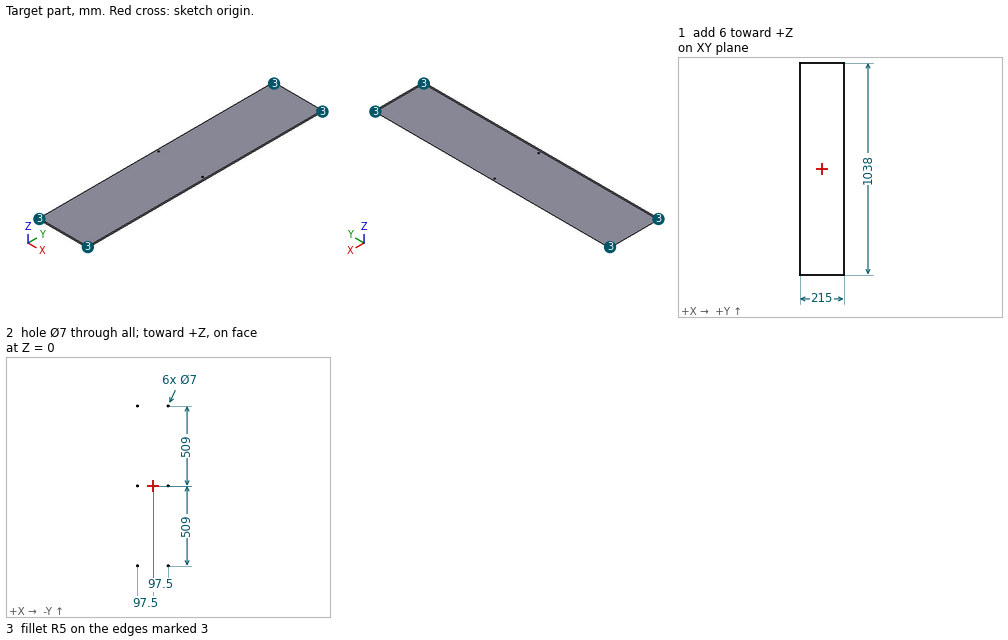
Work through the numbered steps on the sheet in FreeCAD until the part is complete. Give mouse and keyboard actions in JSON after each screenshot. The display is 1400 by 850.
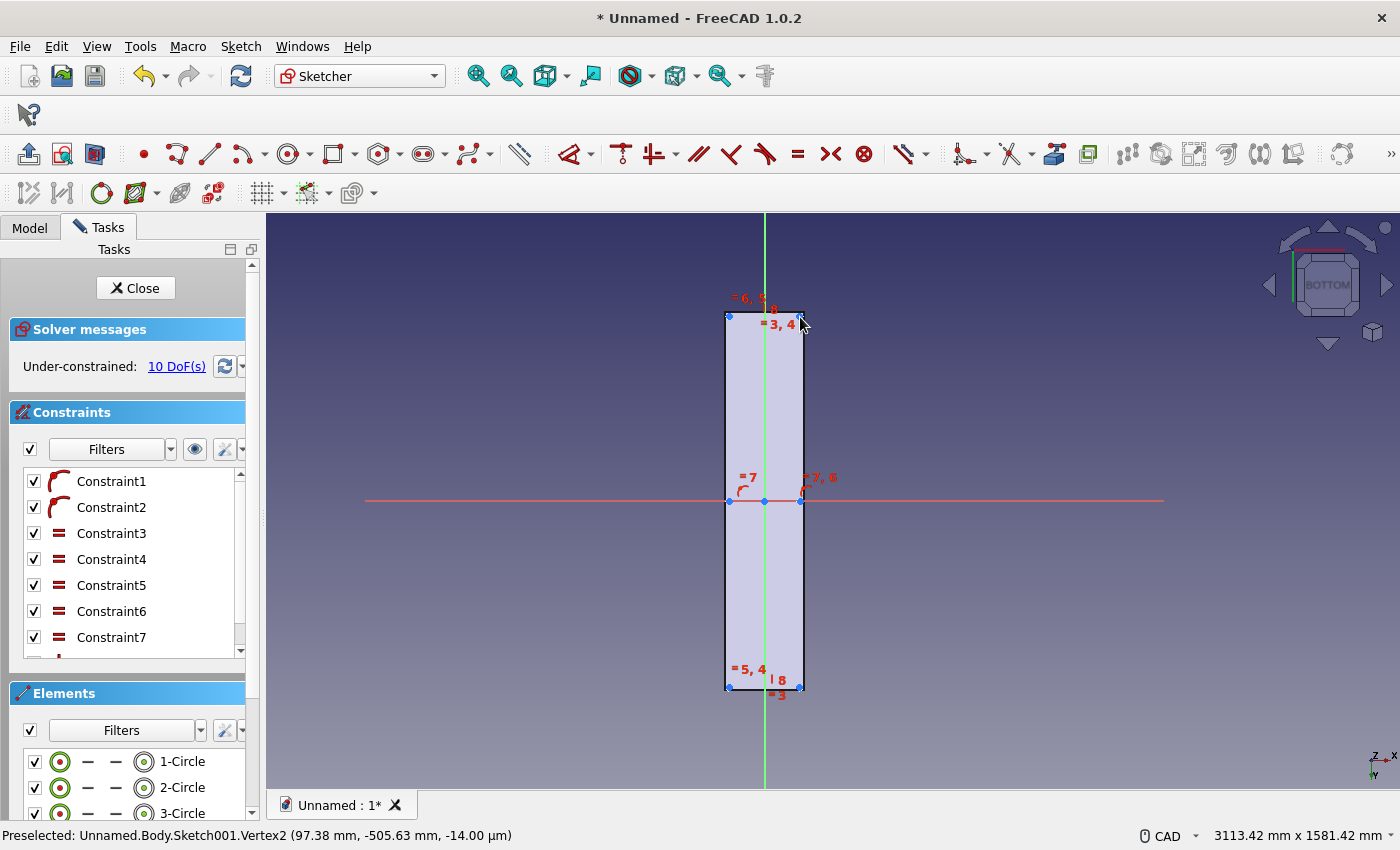
{"action": "left_click", "coordinate": [800, 688]}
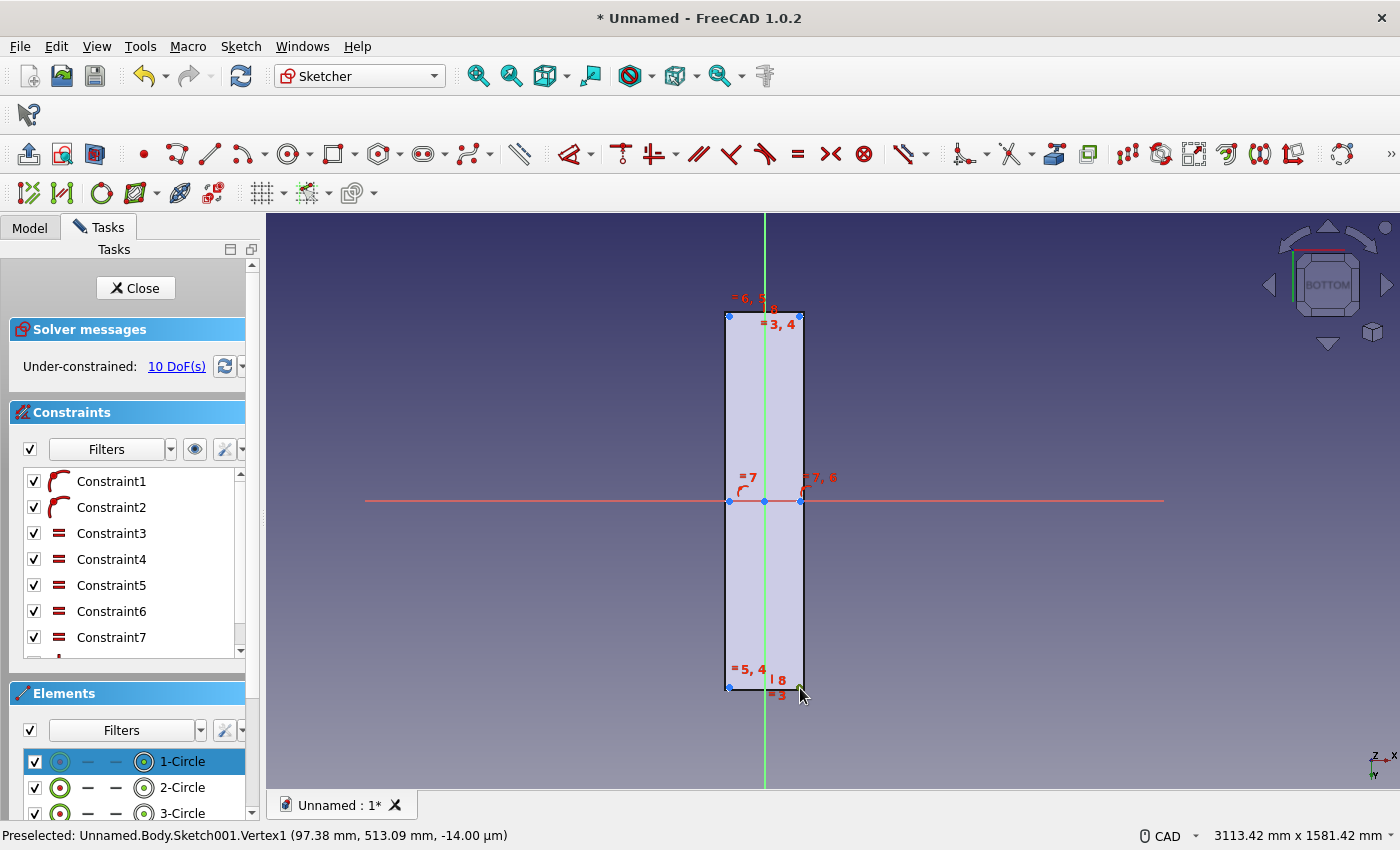
{"action": "left_click", "coordinate": [729, 688]}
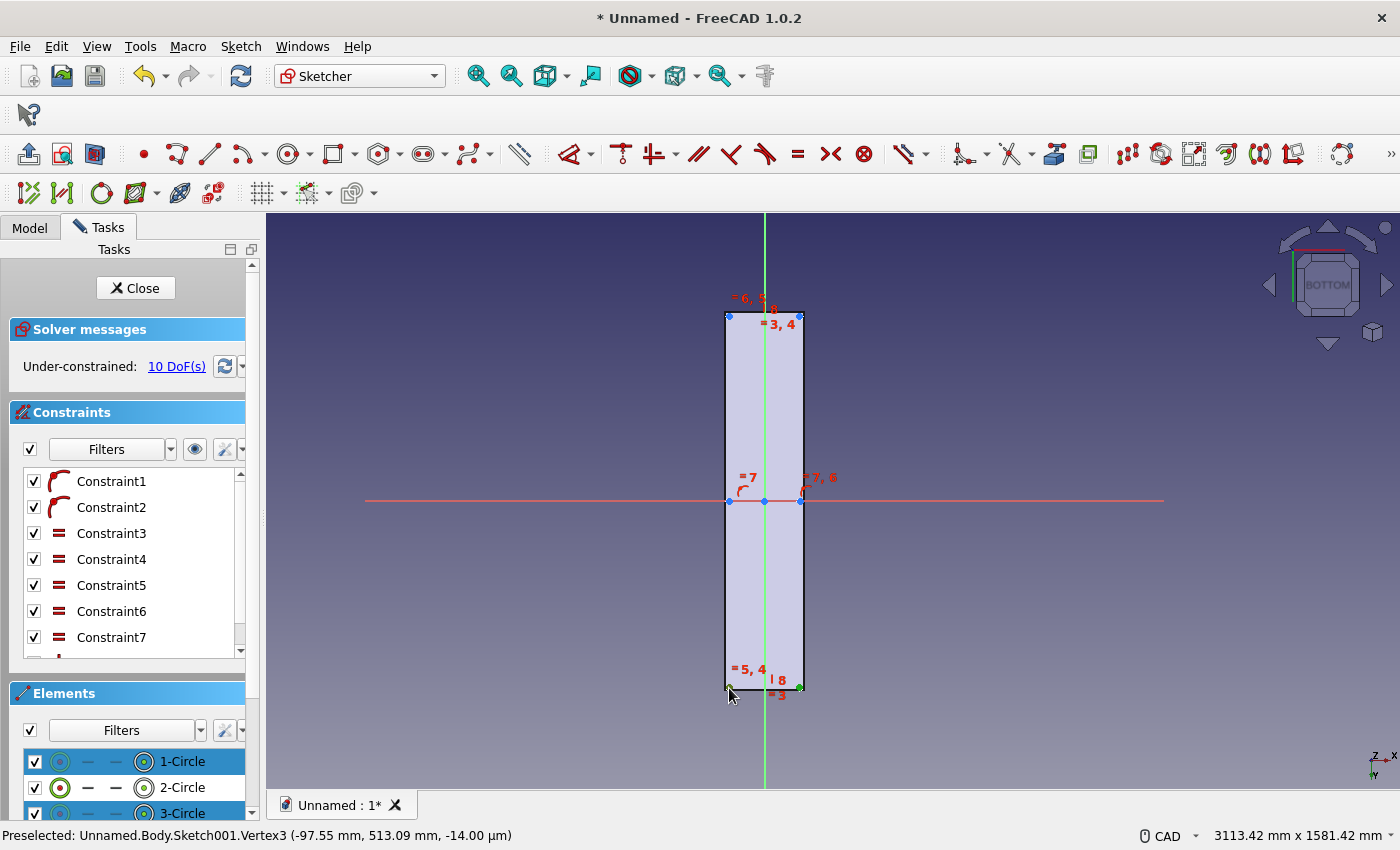
{"action": "left_click", "coordinate": [676, 154]}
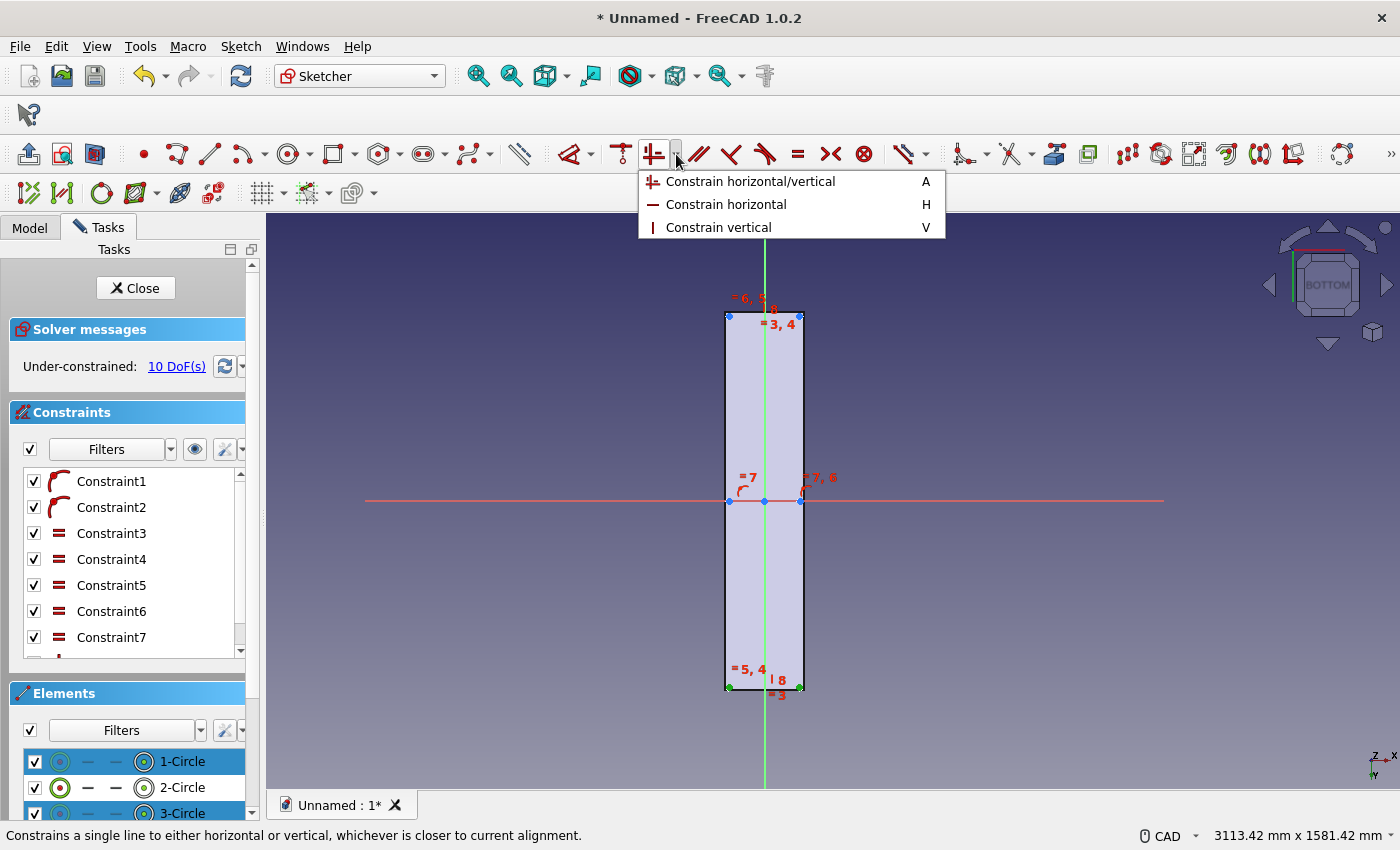
{"action": "left_click", "coordinate": [792, 204]}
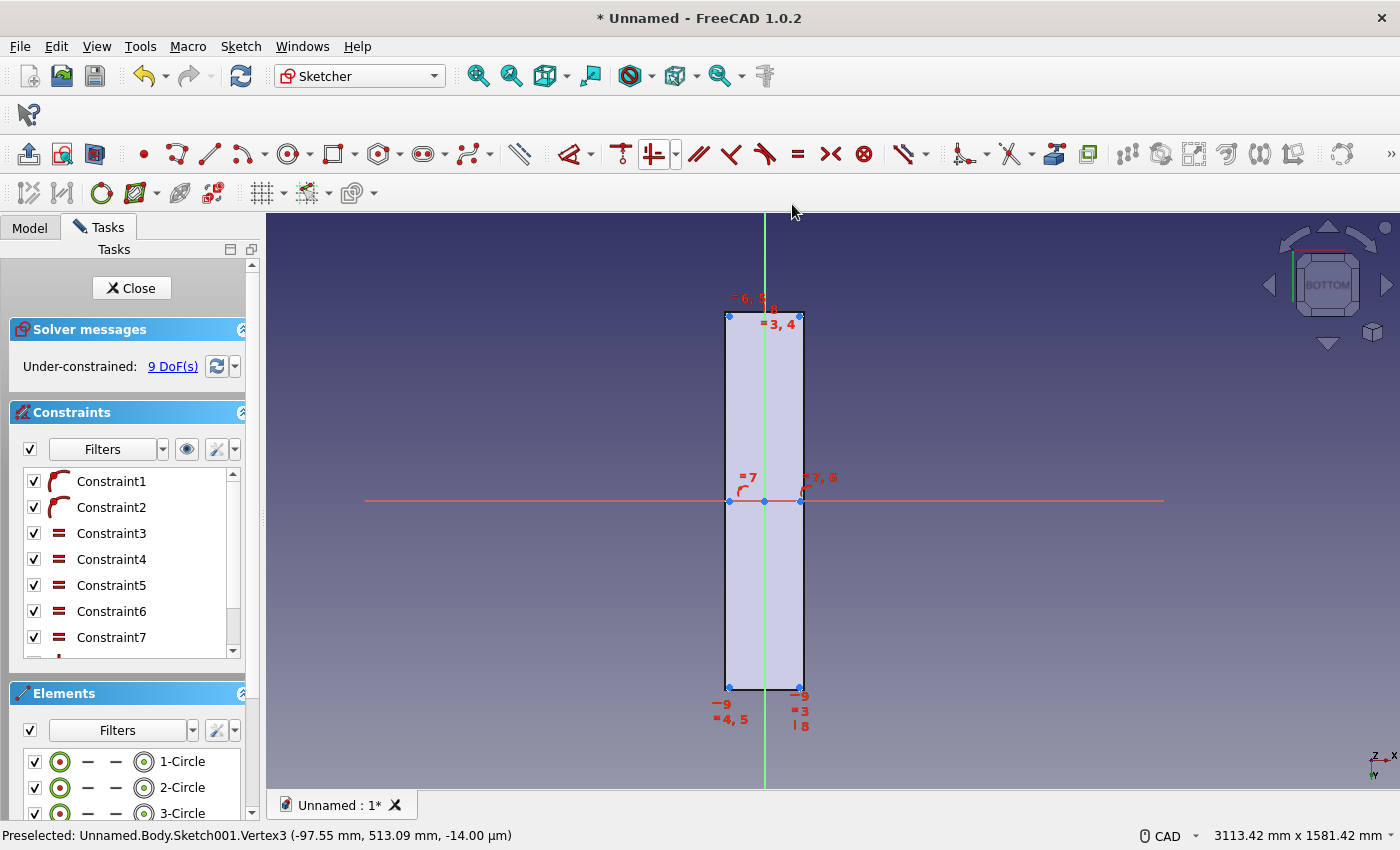
{"action": "left_click", "coordinate": [729, 688]}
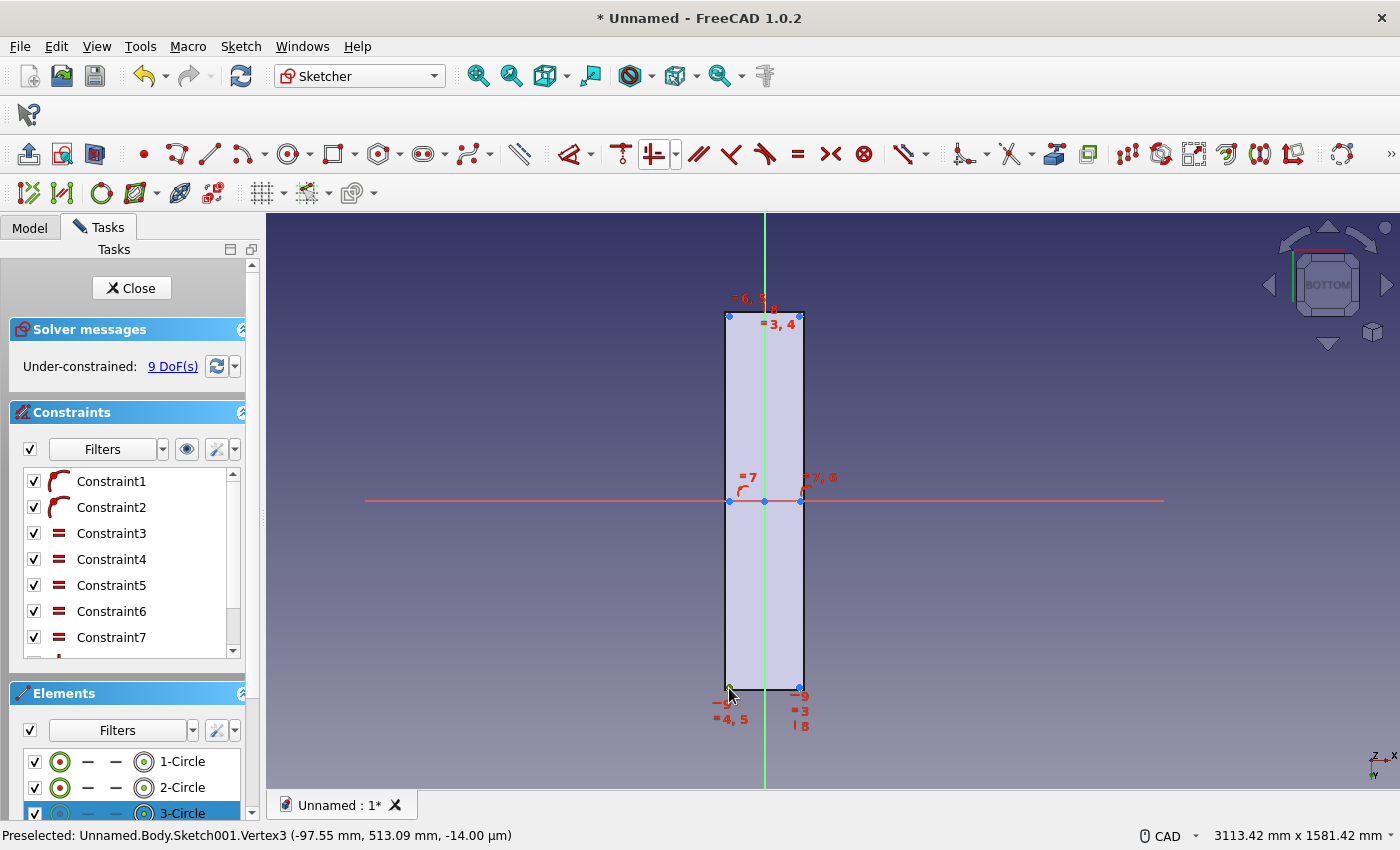
{"action": "left_click", "coordinate": [729, 317]}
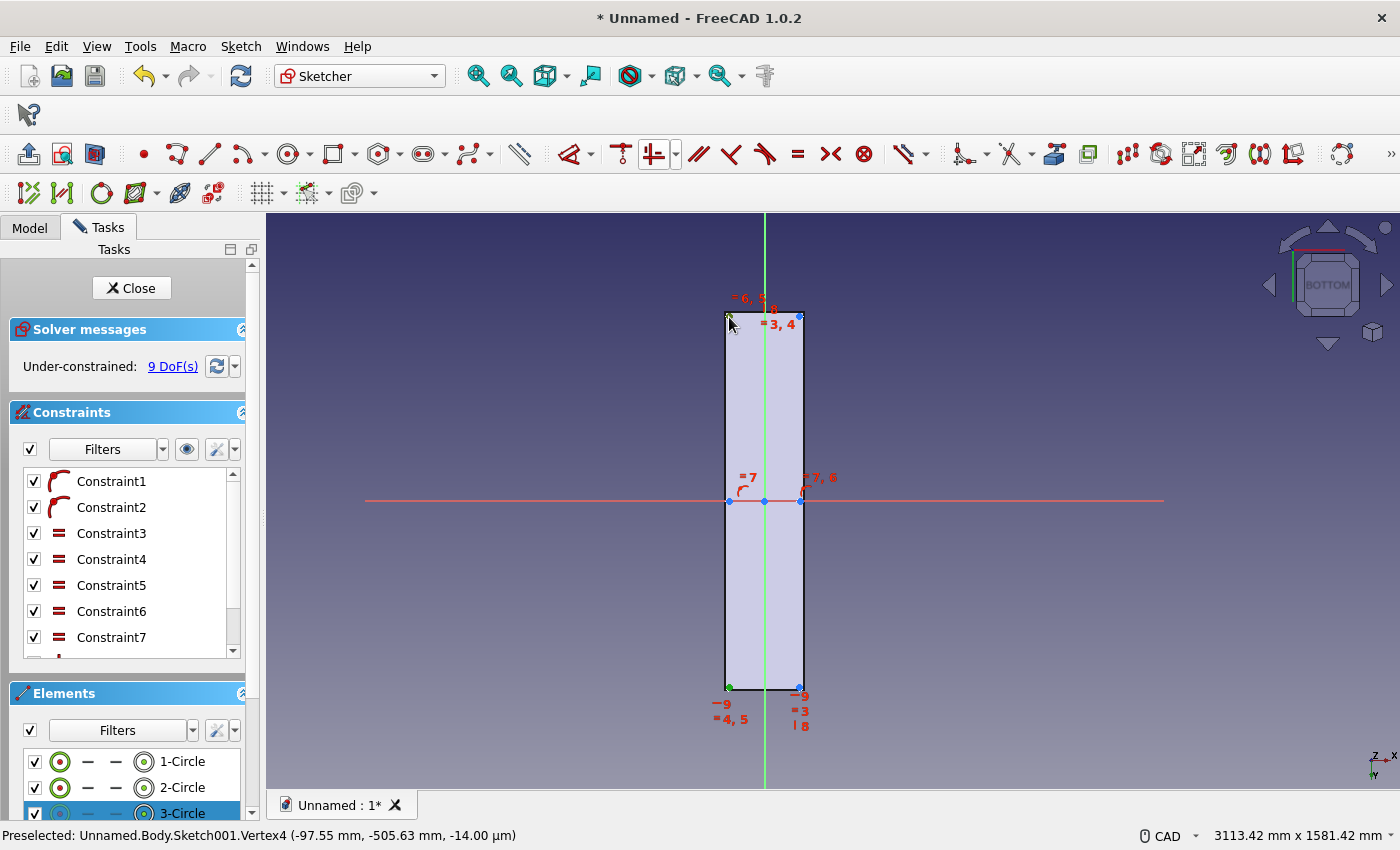
{"action": "left_click", "coordinate": [676, 154]}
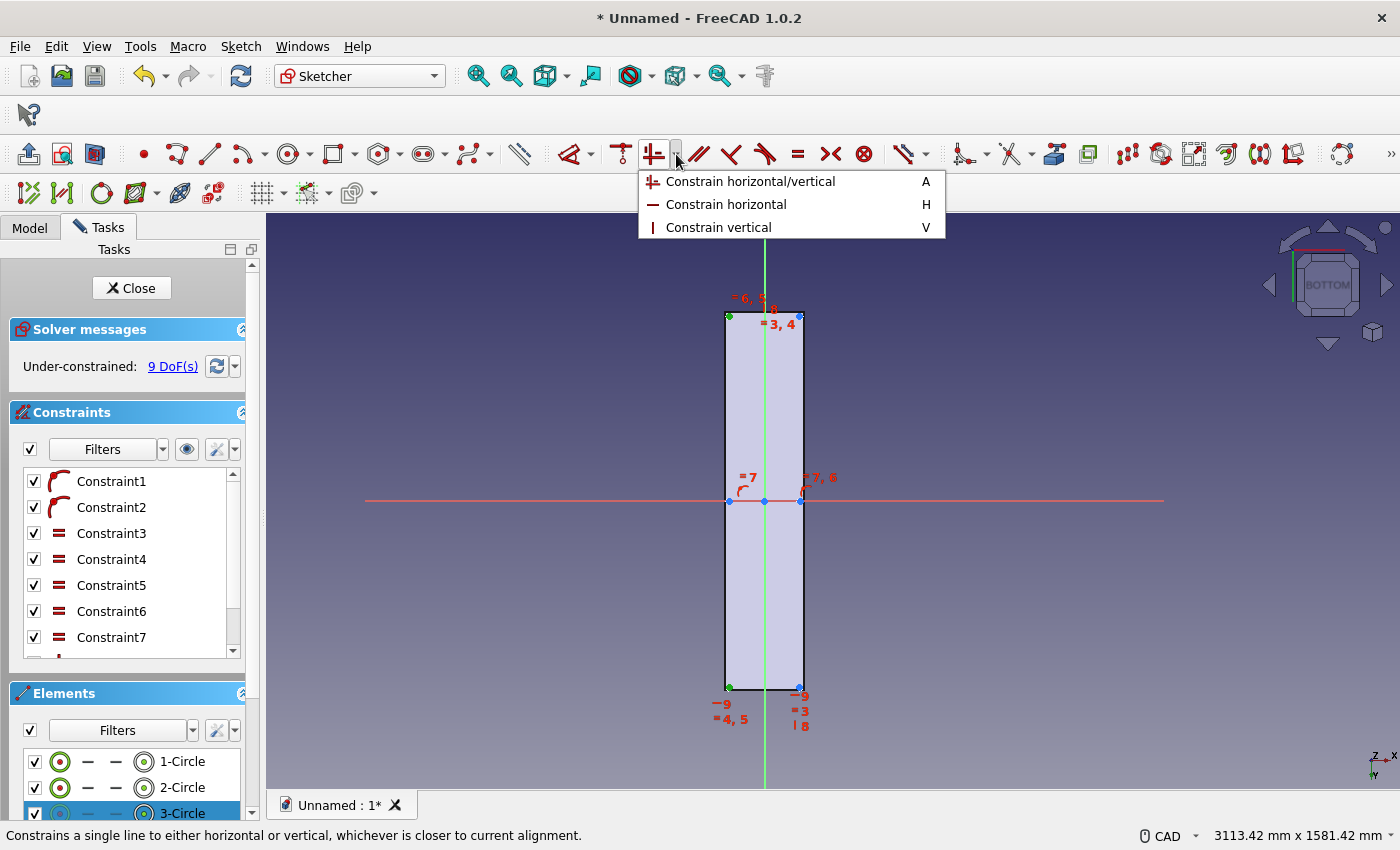
{"action": "left_click", "coordinate": [792, 228]}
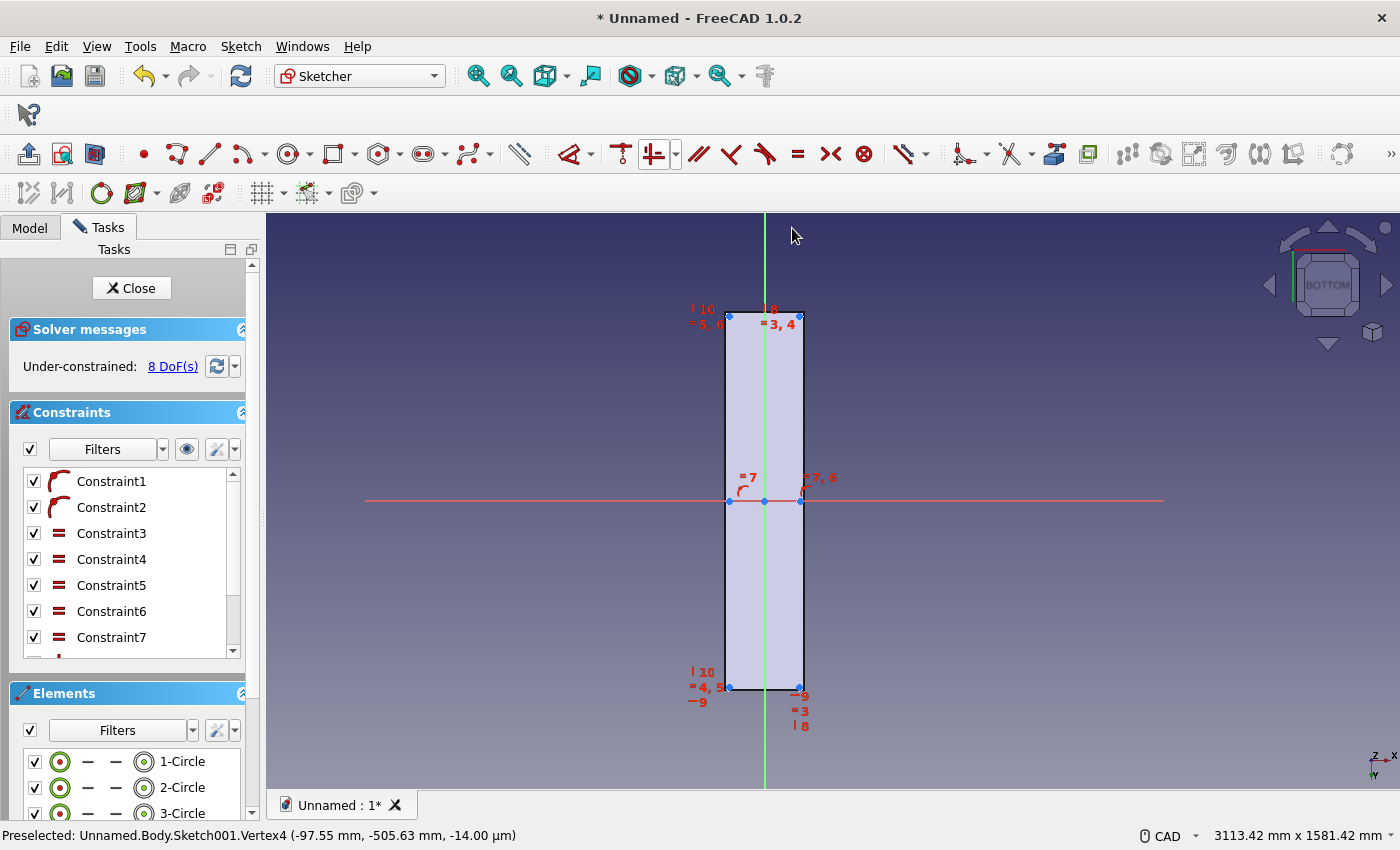
{"action": "left_click", "coordinate": [800, 317]}